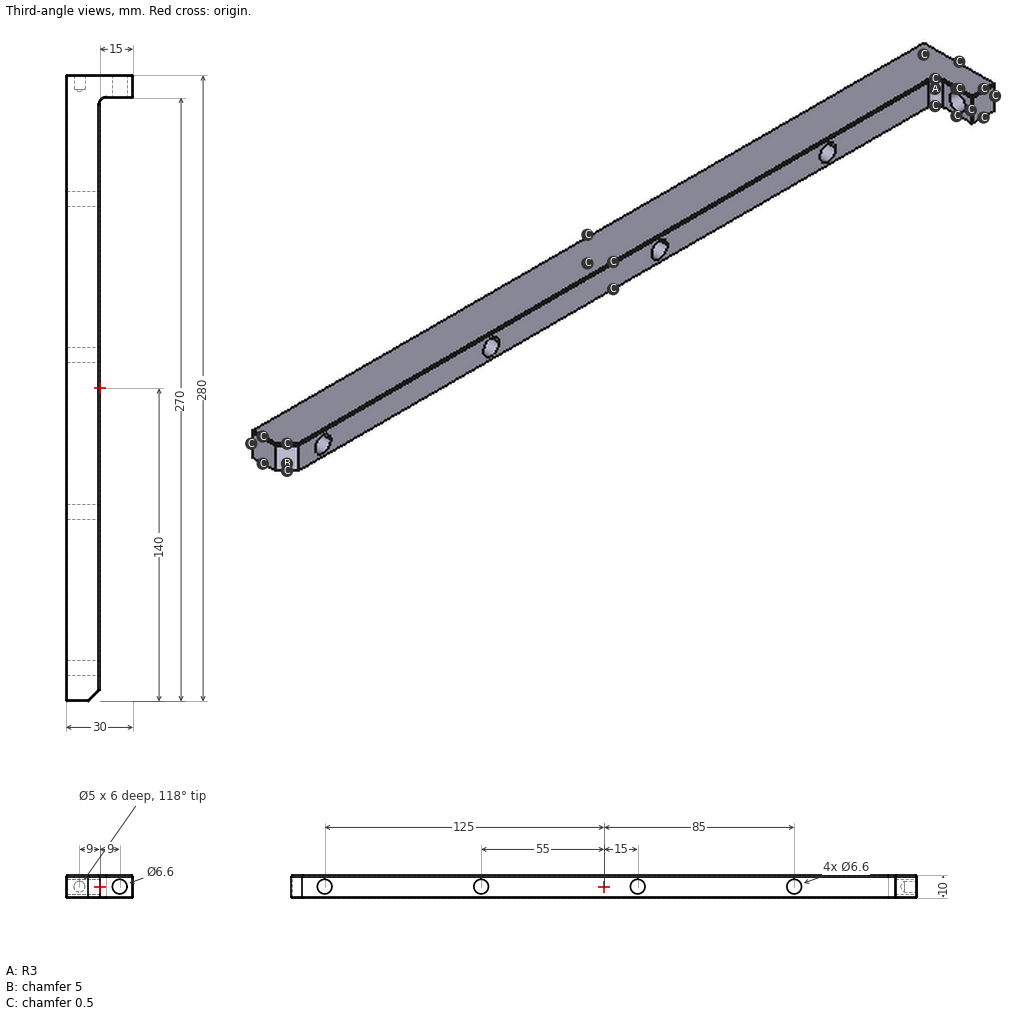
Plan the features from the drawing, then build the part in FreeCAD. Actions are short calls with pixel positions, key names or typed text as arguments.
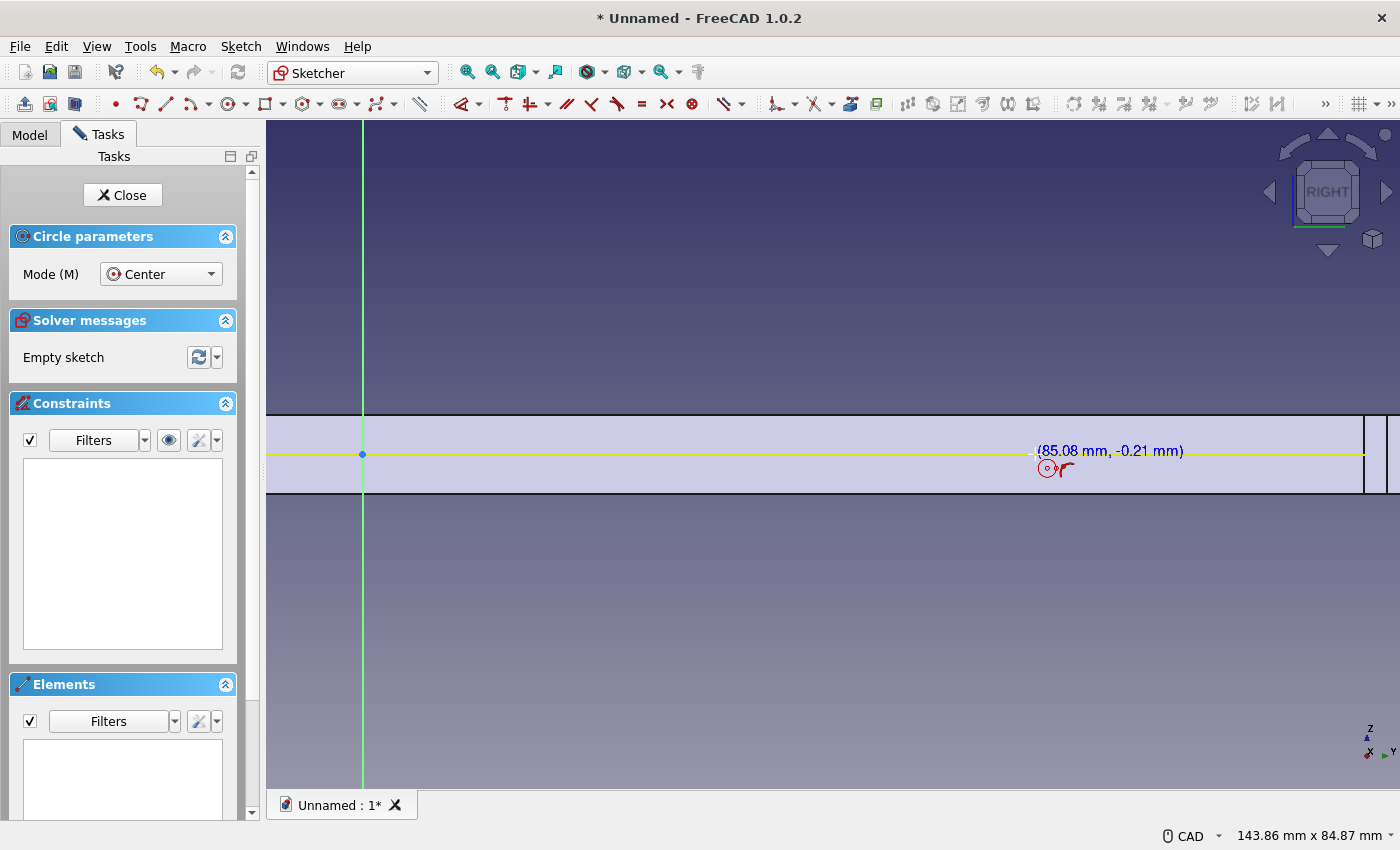
click(1033, 454)
click(1051, 436)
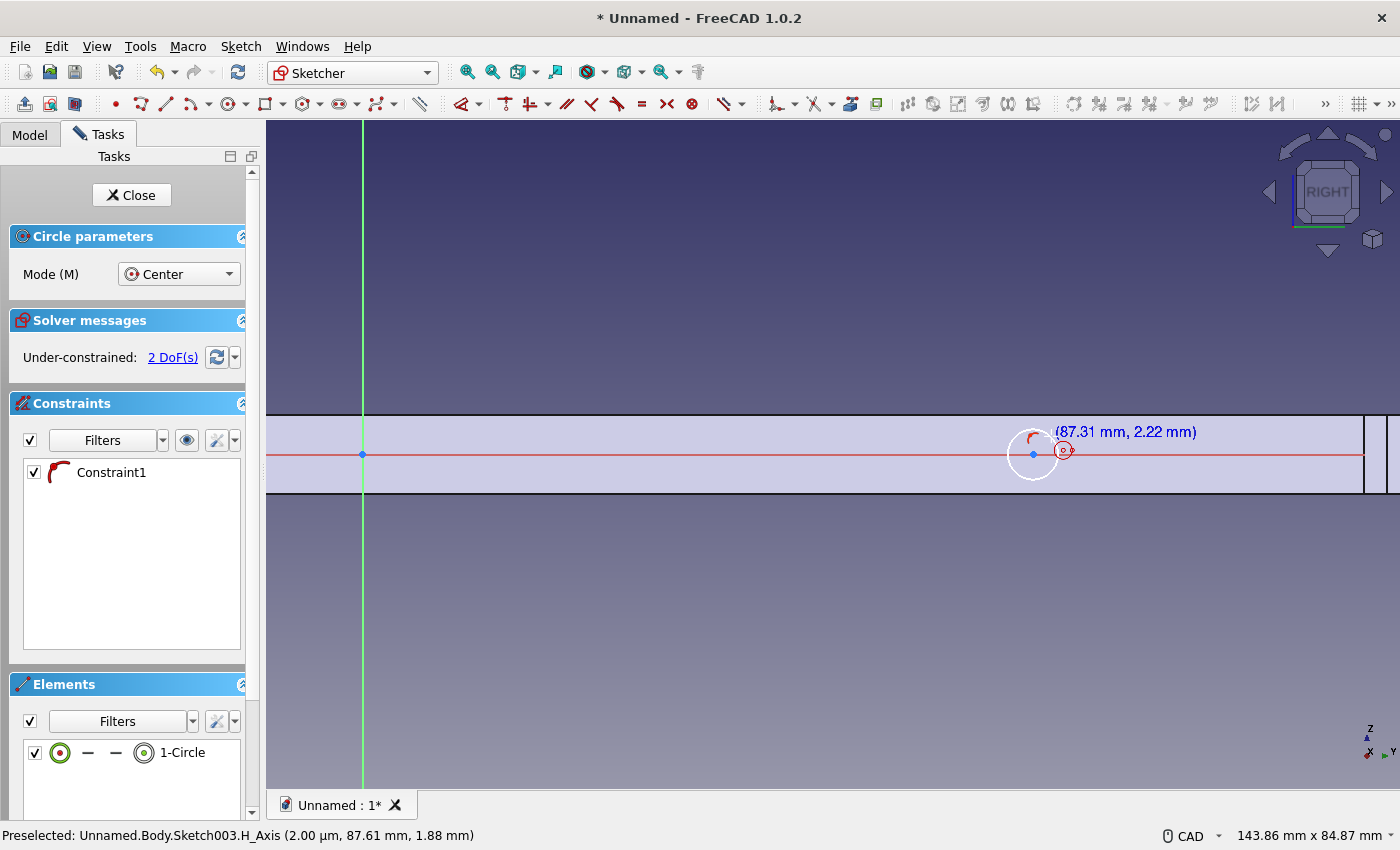
click(481, 454)
click(499, 436)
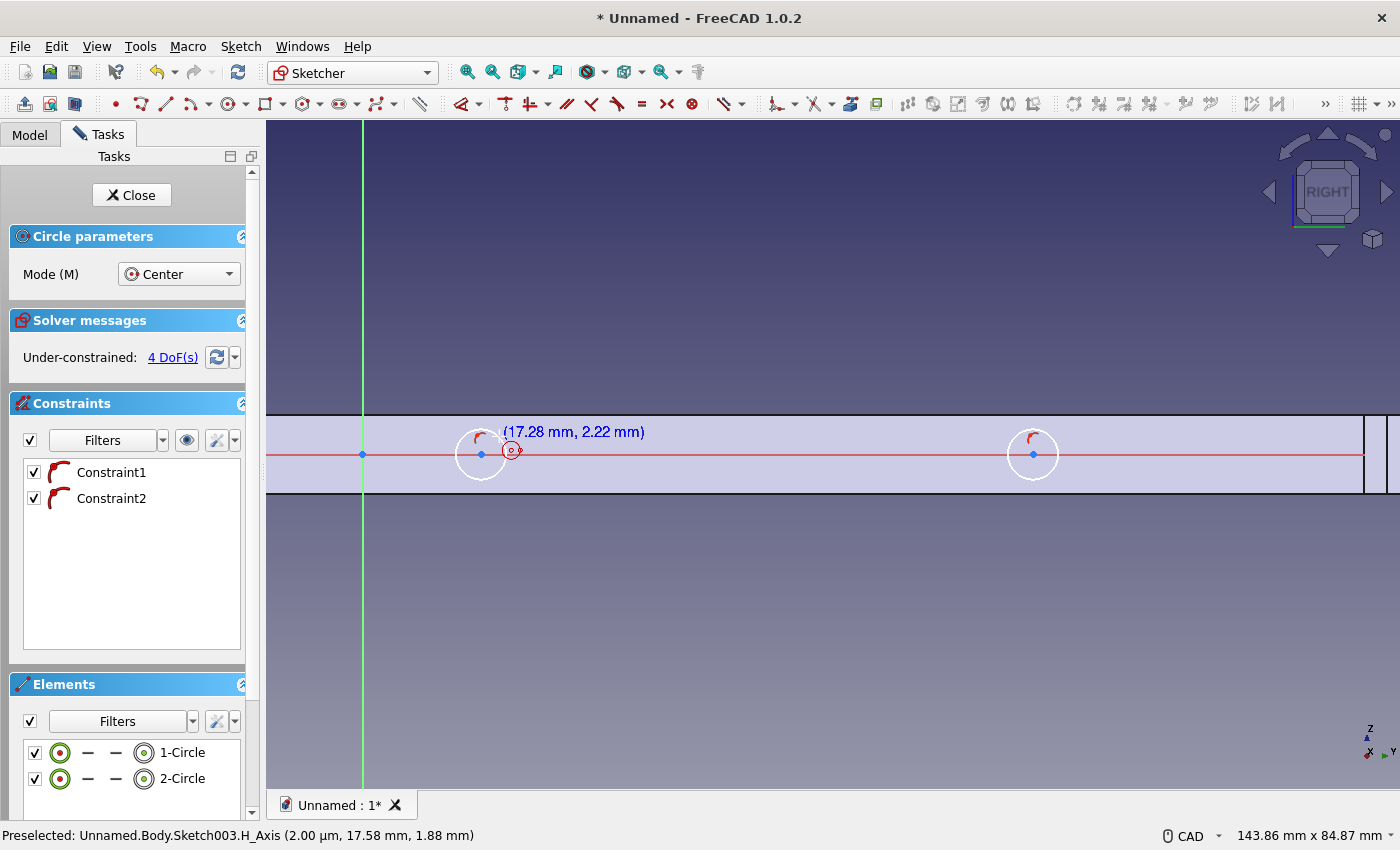
scroll(1090, 455, down, 5)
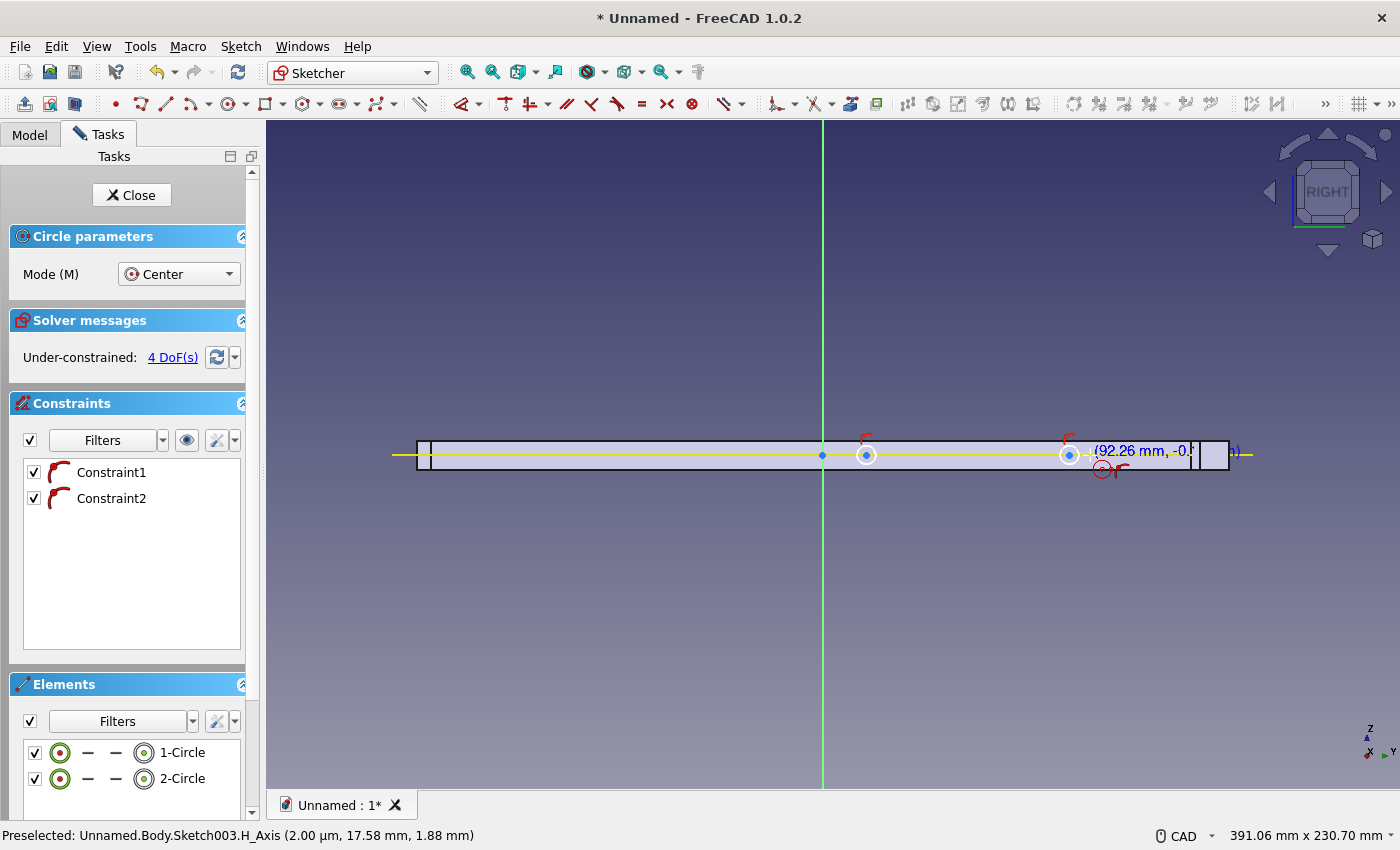
scroll(663, 455, up, 5)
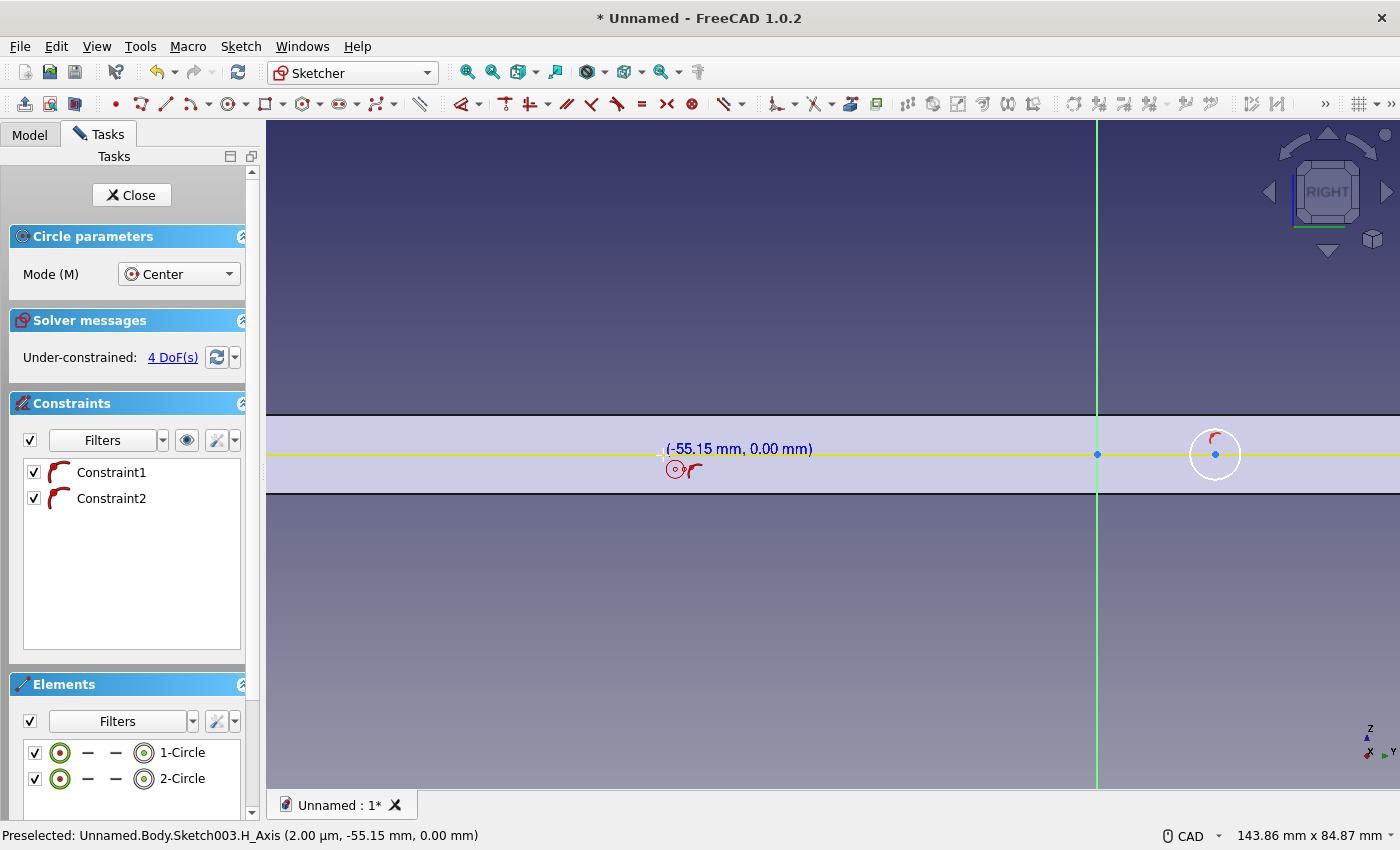
click(664, 454)
click(682, 436)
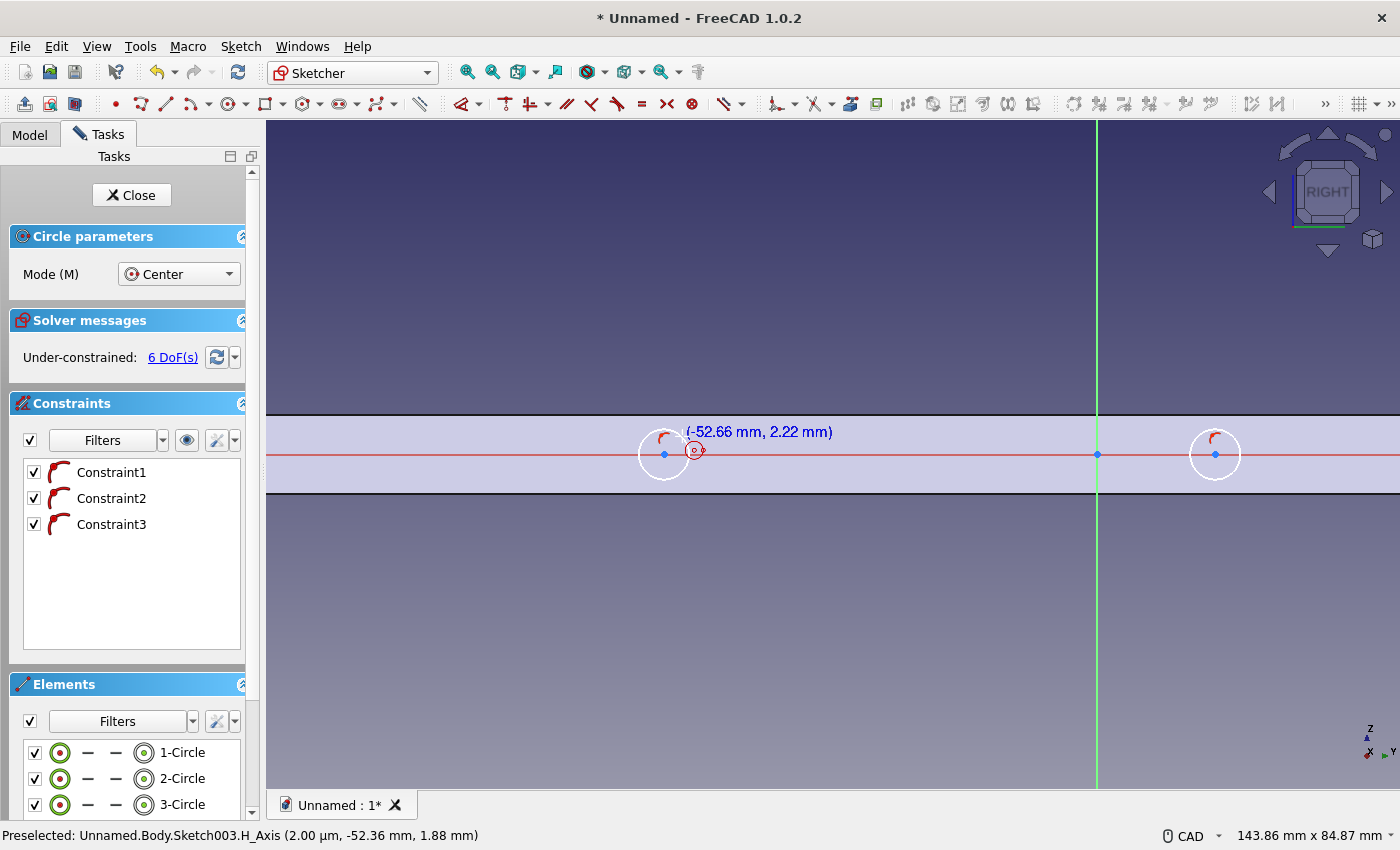
scroll(663, 455, down, 5)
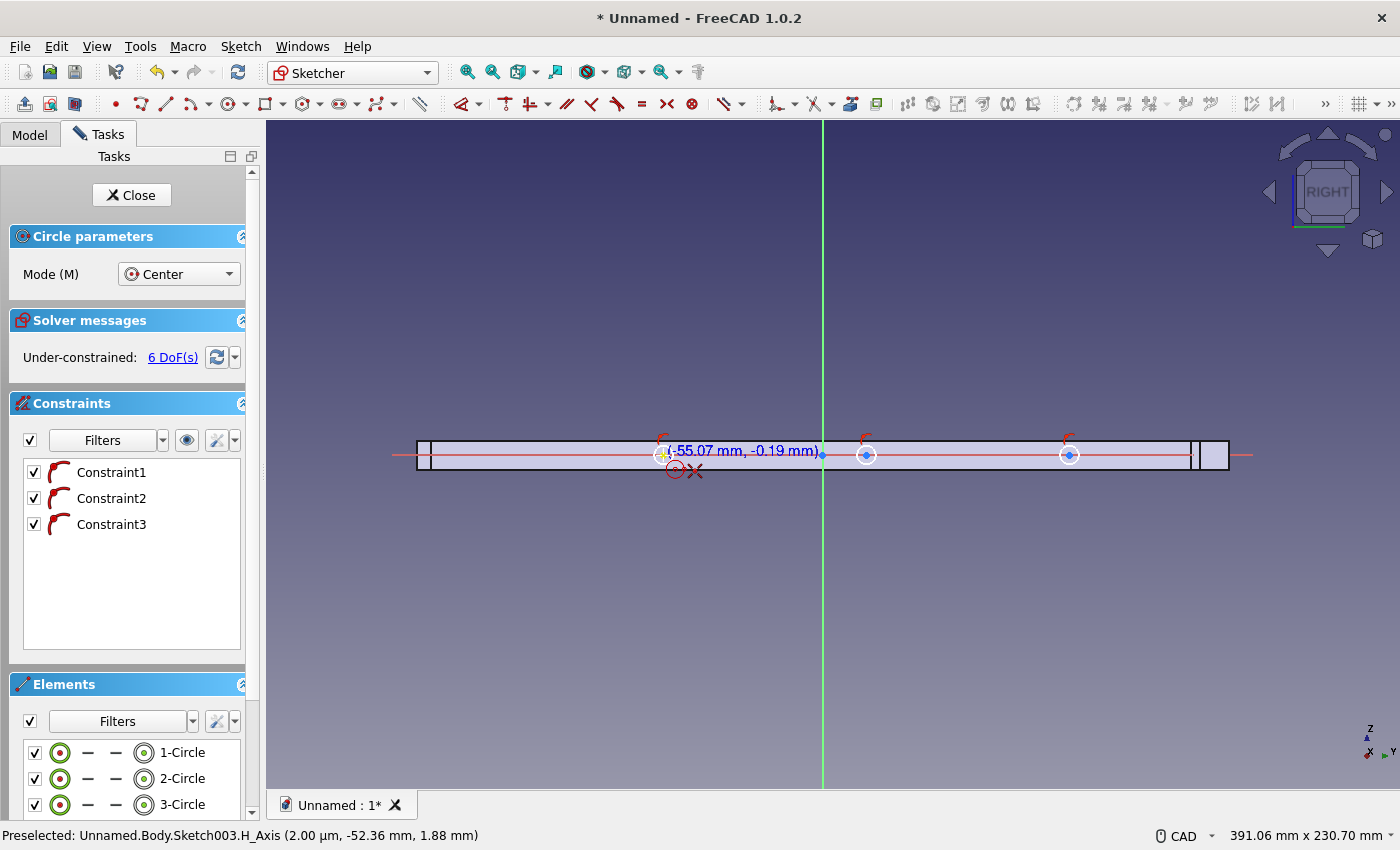
scroll(460, 455, up, 5)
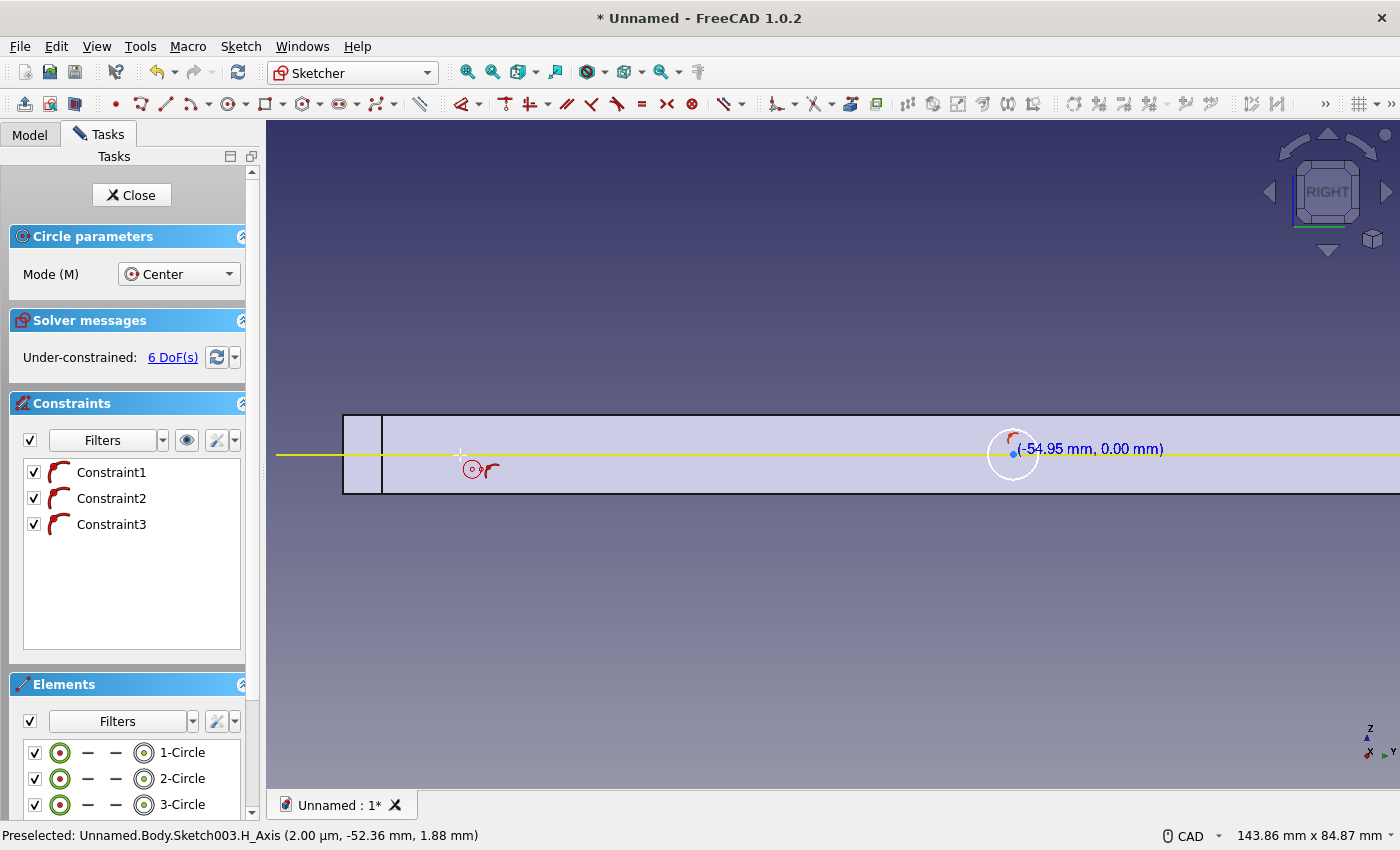
click(461, 454)
click(479, 436)
key(Escape)